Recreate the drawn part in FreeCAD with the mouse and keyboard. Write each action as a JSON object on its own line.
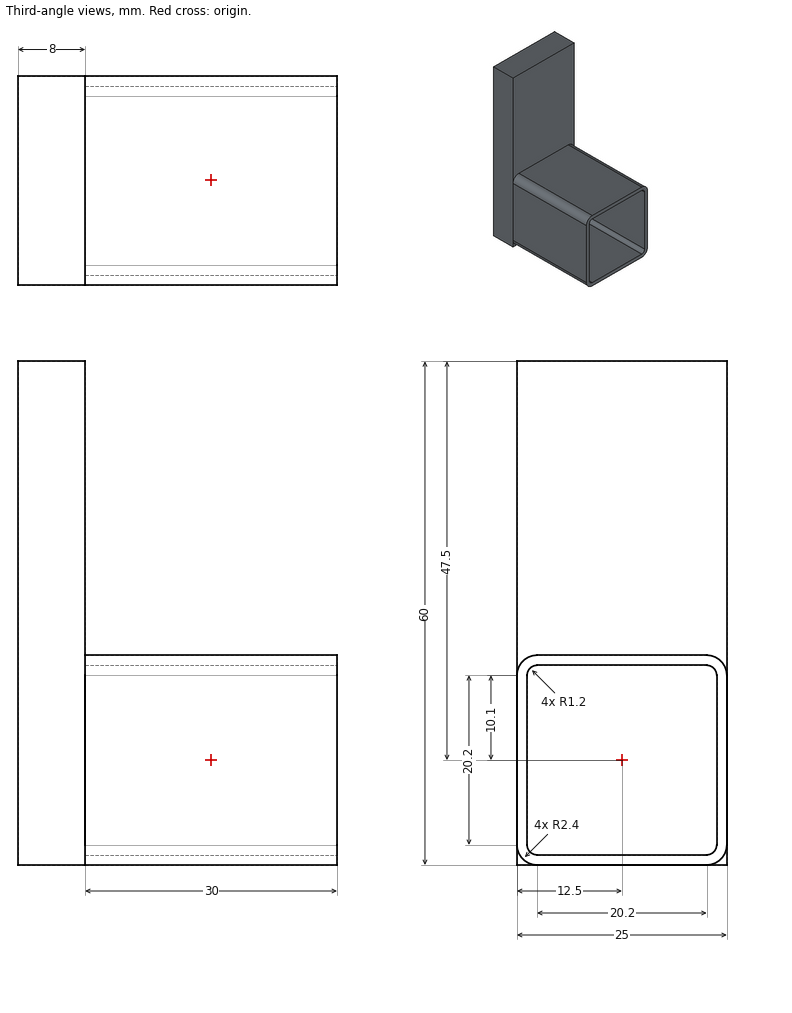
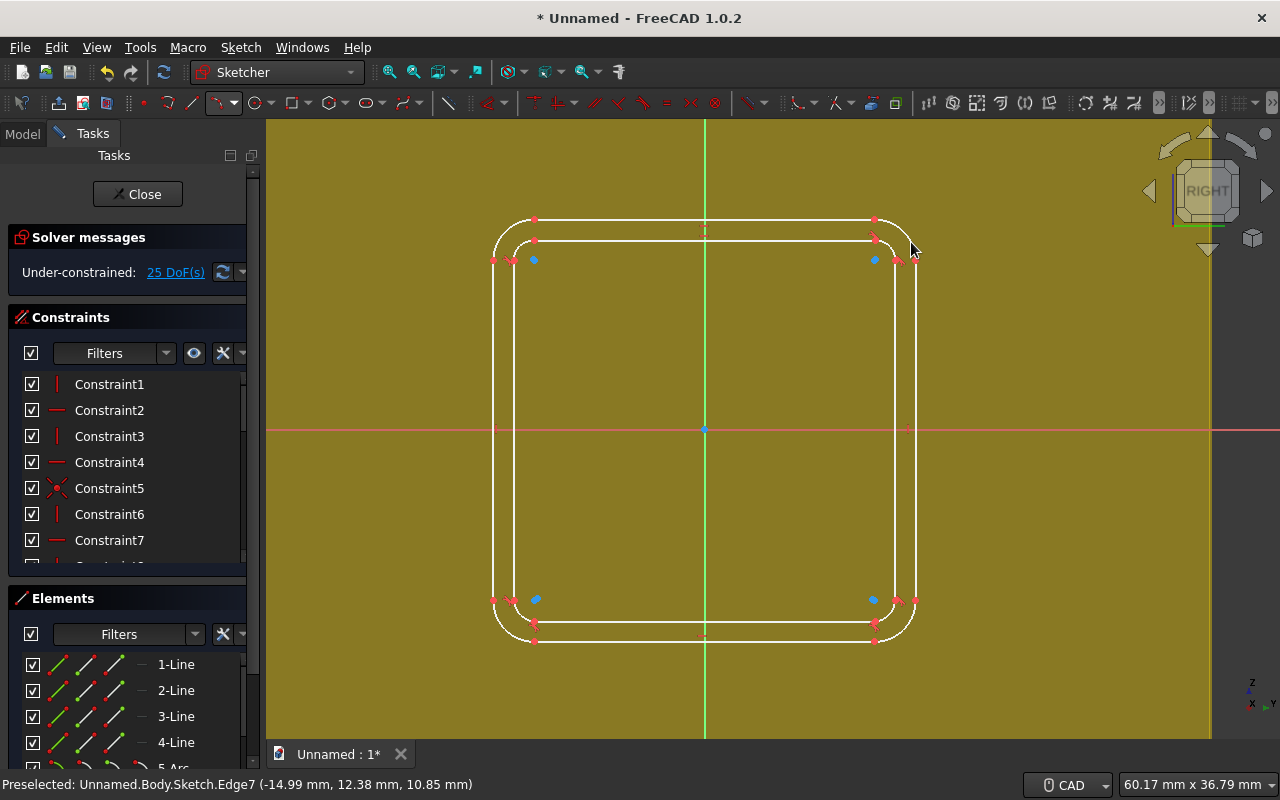
{"action": "left_click", "coordinate": [773, 220]}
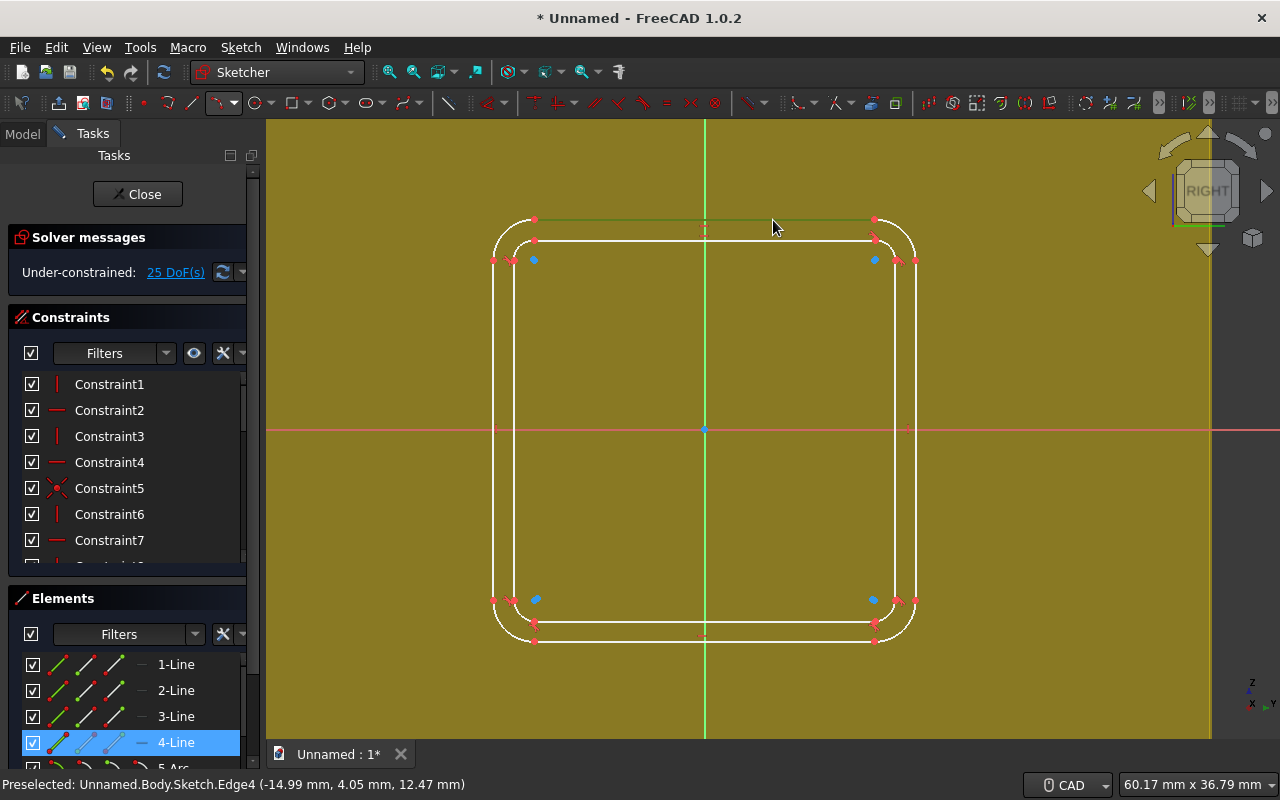
{"action": "left_click", "coordinate": [516, 224]}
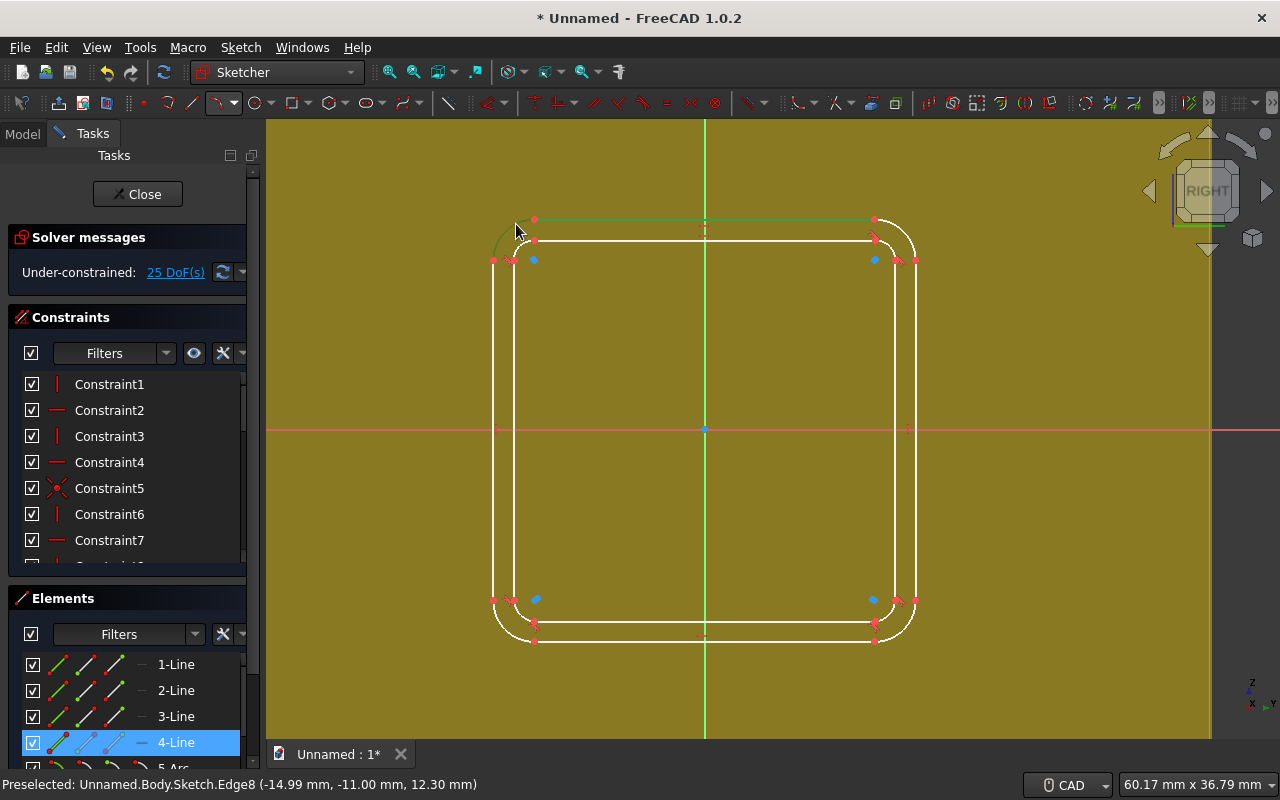
{"action": "key", "text": "t"}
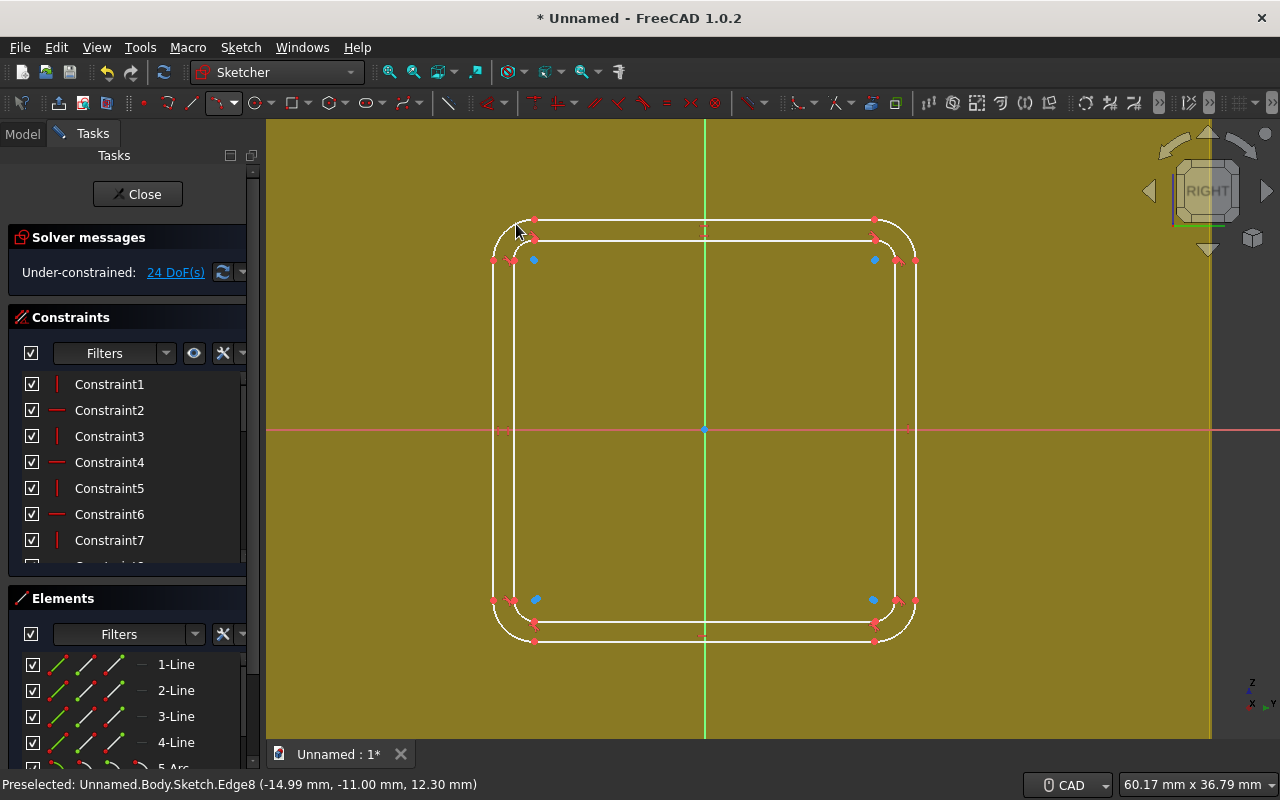
{"action": "left_click", "coordinate": [514, 499]}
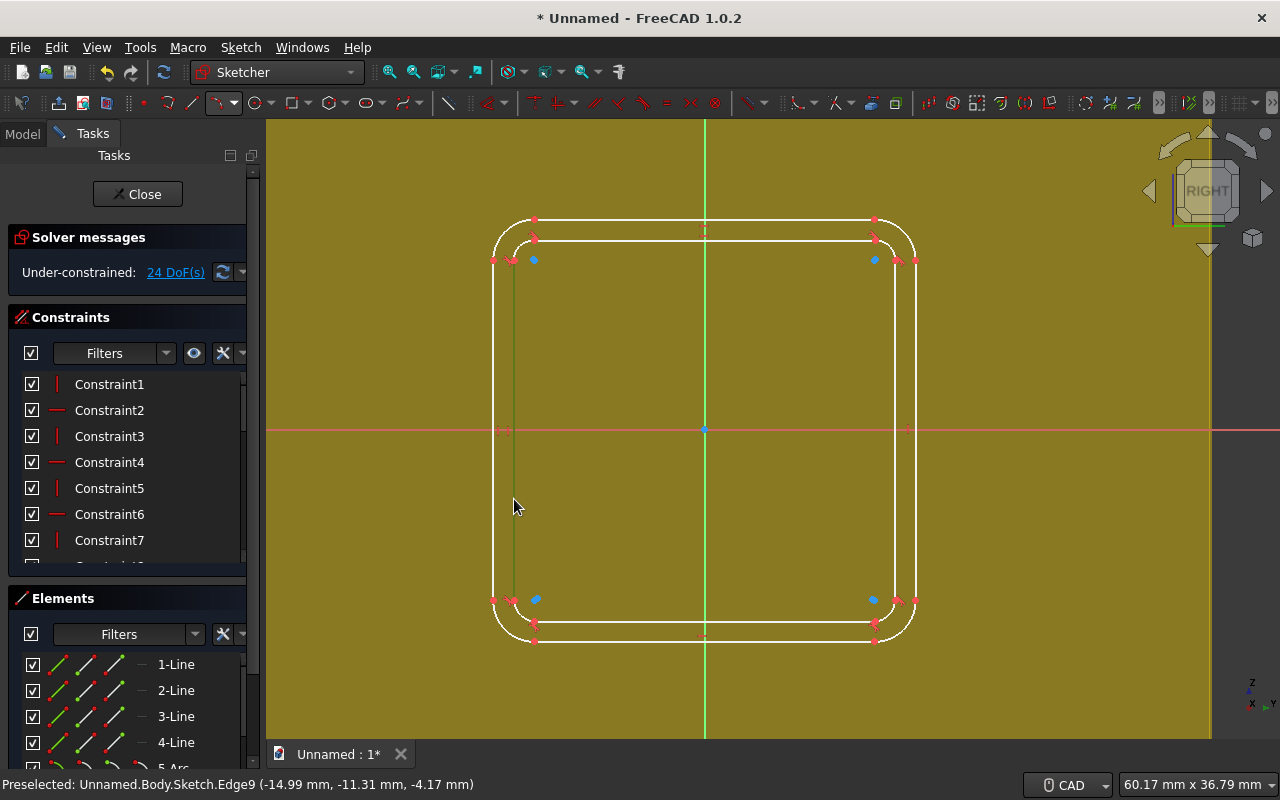
{"action": "scroll", "coordinate": [525, 243], "scroll_direction": "up", "scroll_amount": 2}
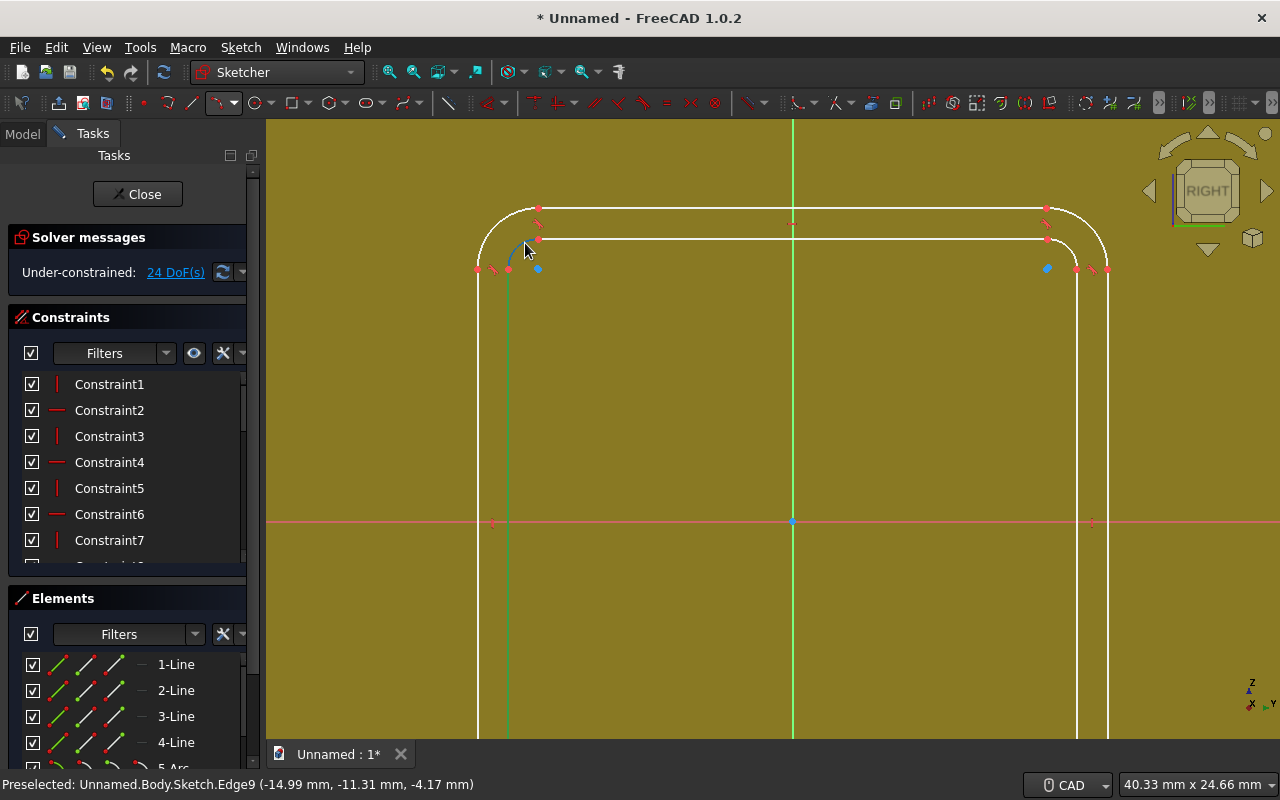
{"action": "left_click", "coordinate": [525, 242]}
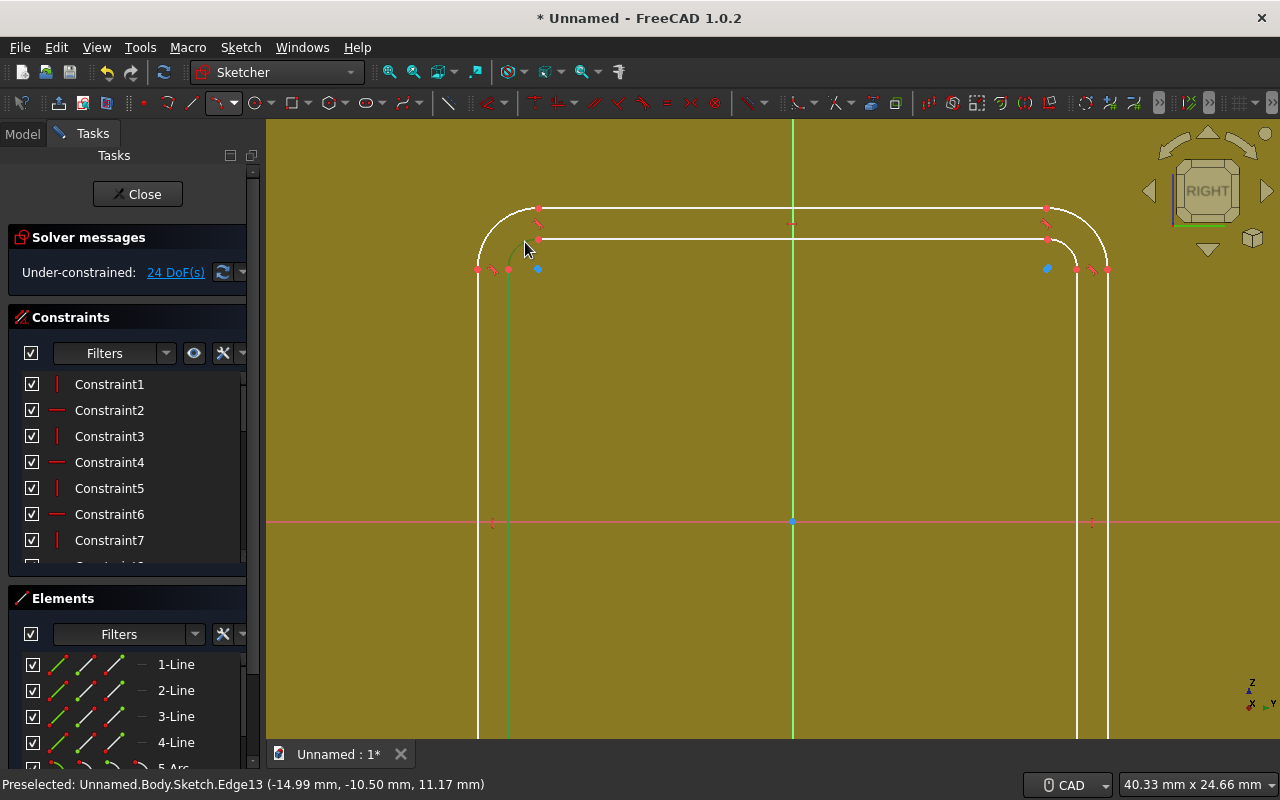
{"action": "key", "text": "t"}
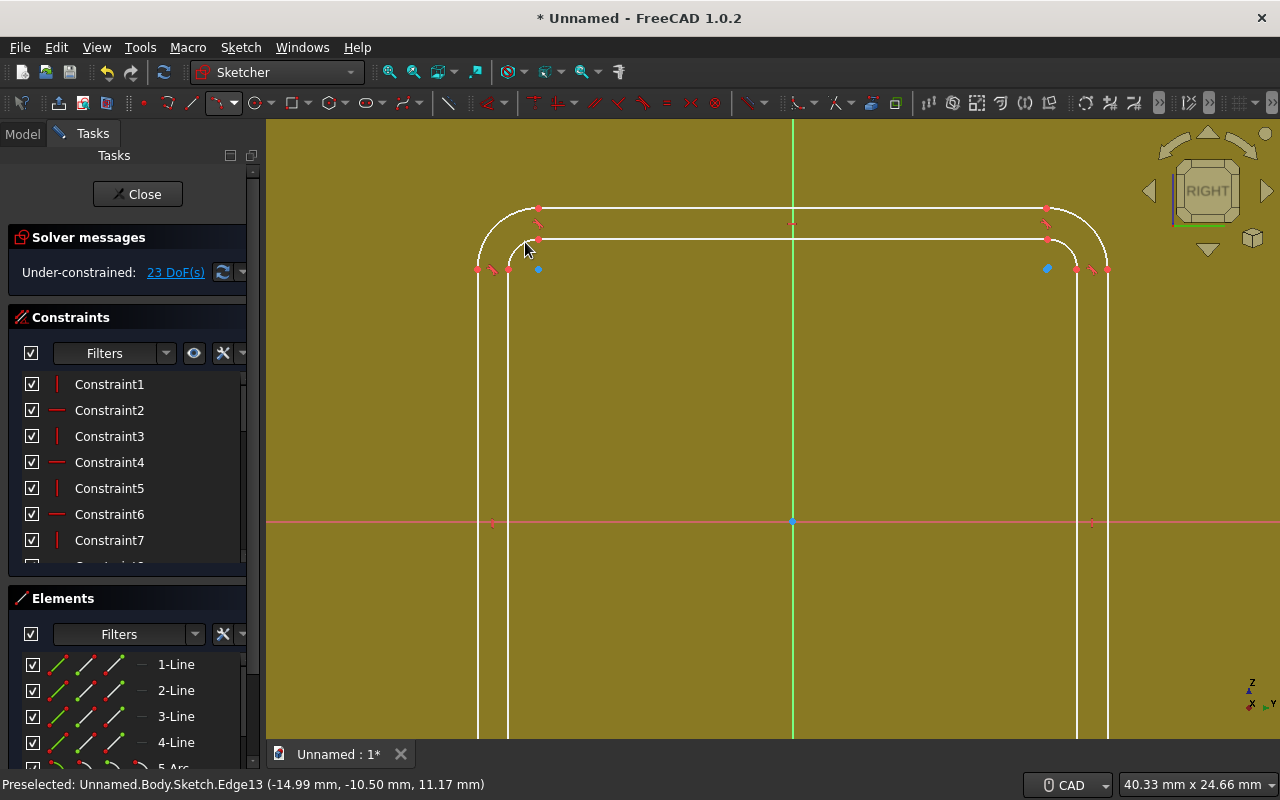
{"action": "left_click", "coordinate": [508, 624]}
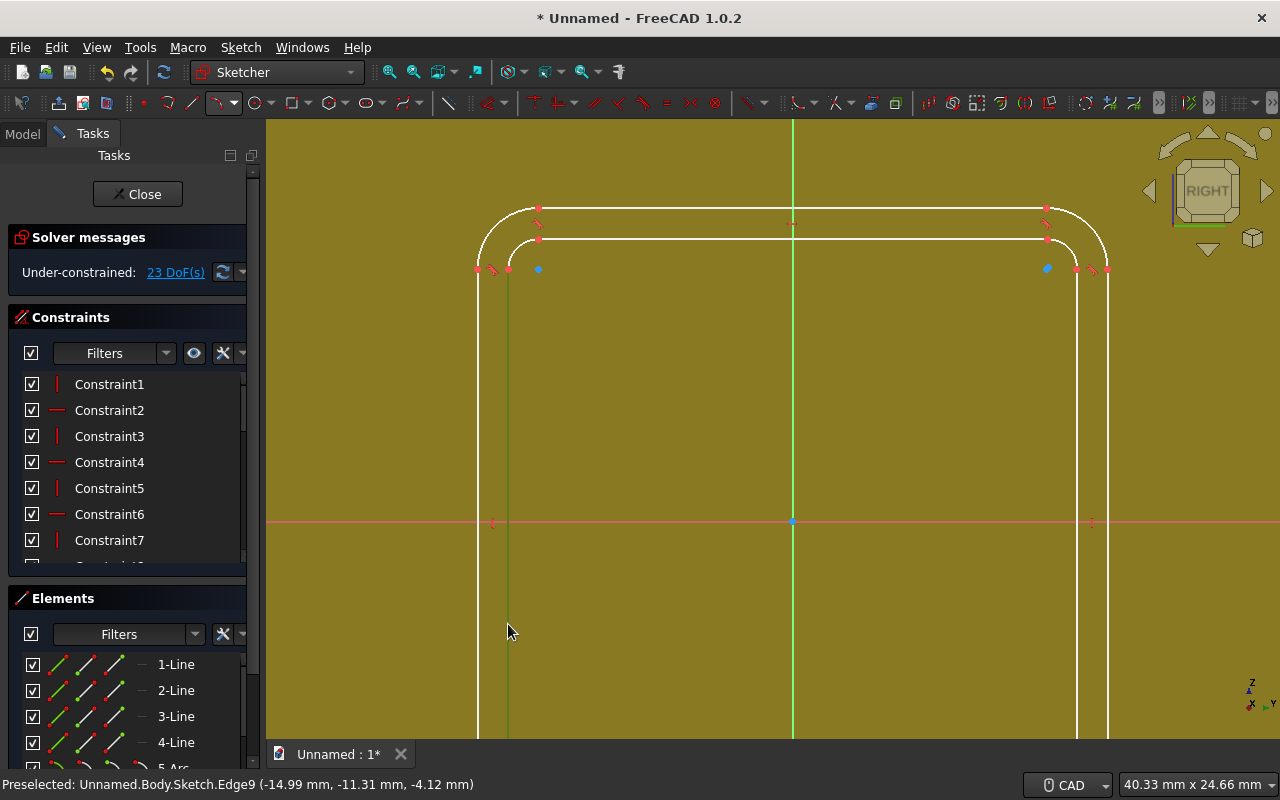
{"action": "scroll", "coordinate": [525, 241], "scroll_direction": "down", "scroll_amount": 2}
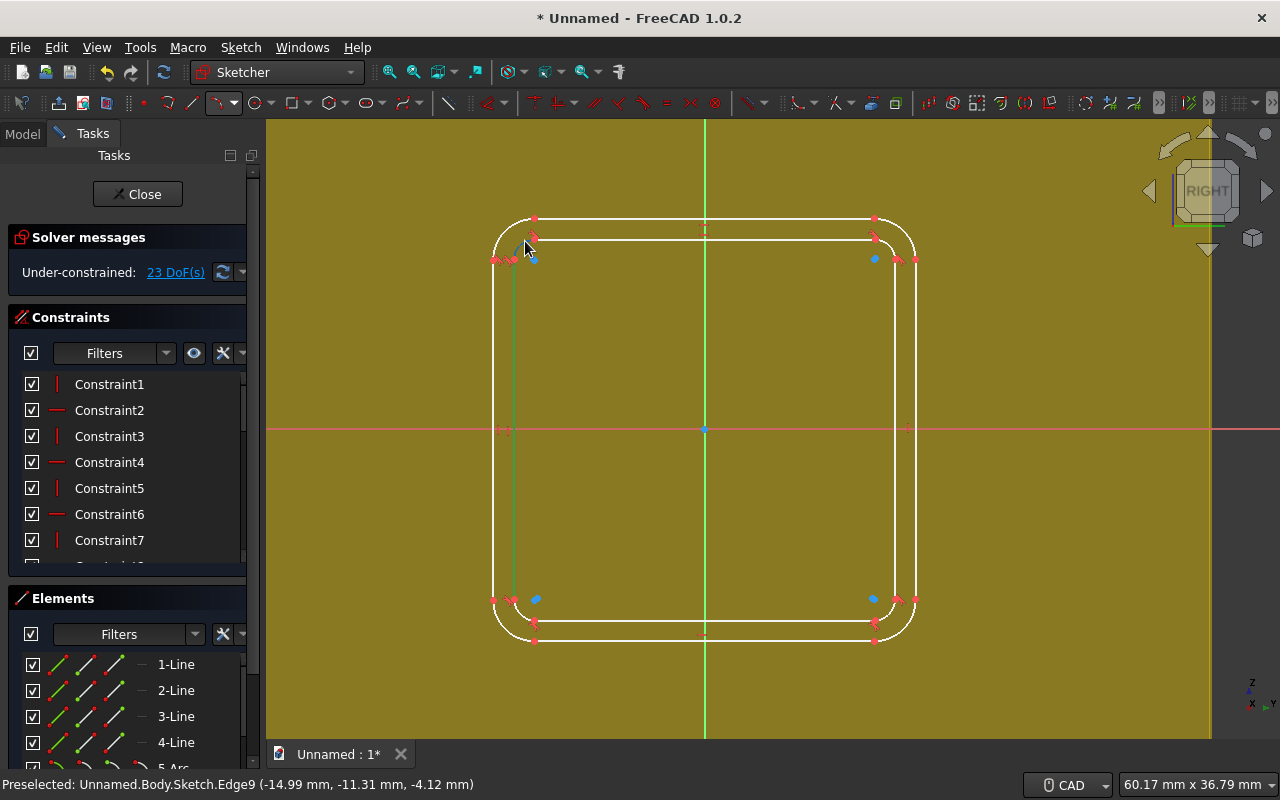
{"action": "scroll", "coordinate": [517, 609], "scroll_direction": "up", "scroll_amount": 2}